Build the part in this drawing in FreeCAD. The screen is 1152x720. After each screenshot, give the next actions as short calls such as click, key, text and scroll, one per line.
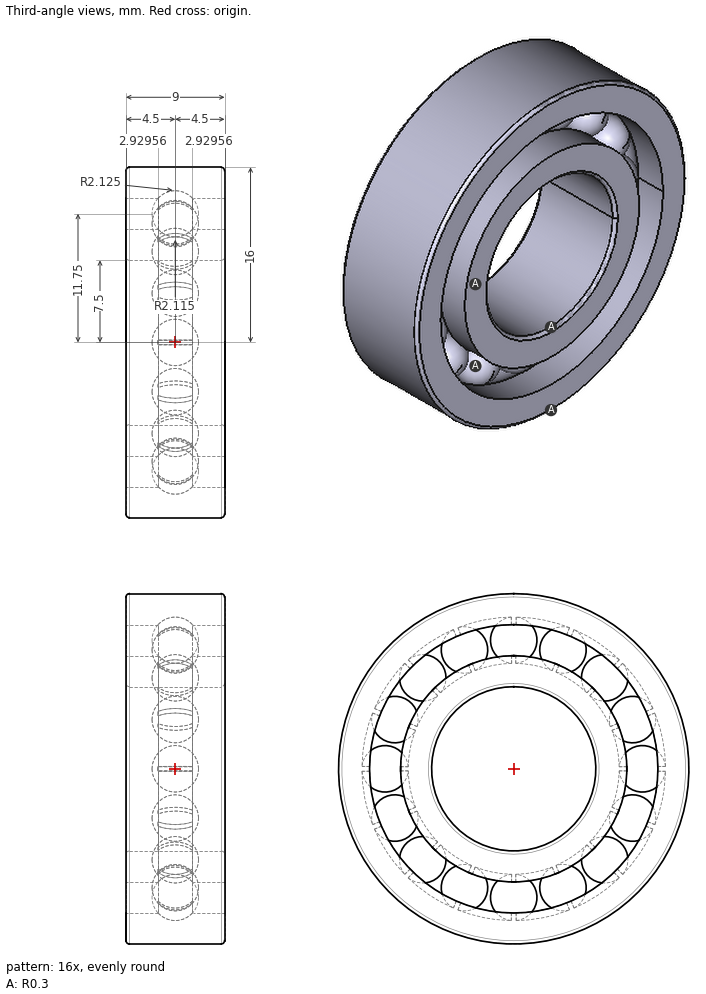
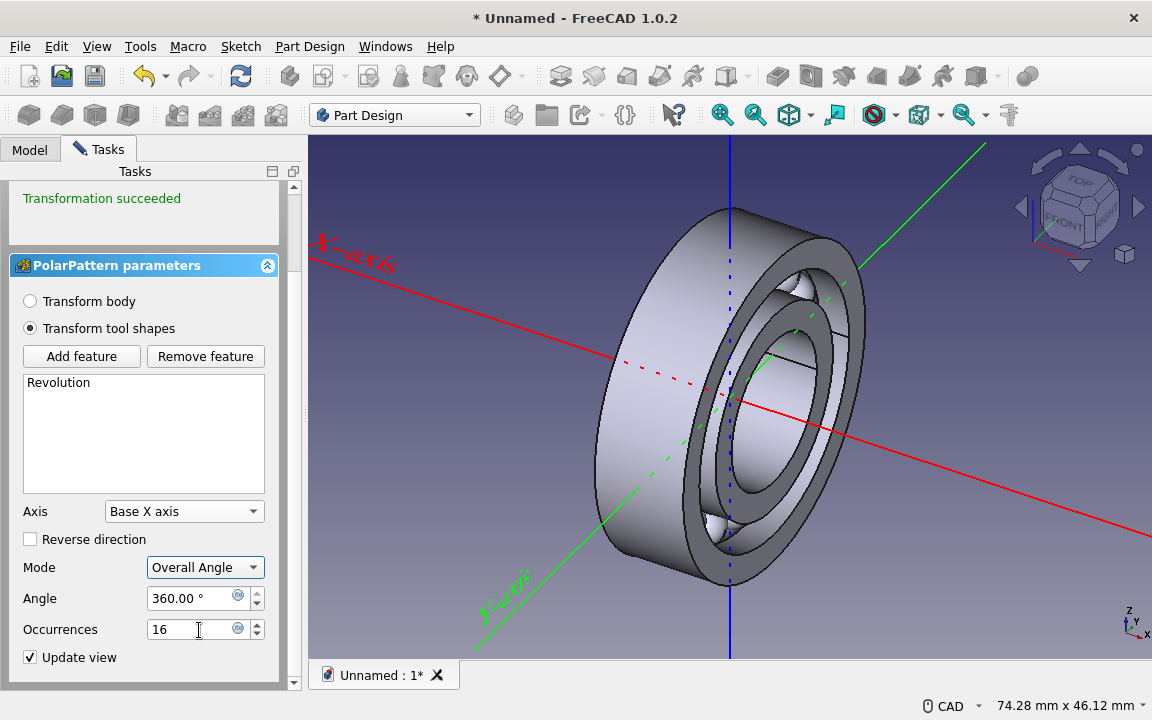
scroll(294, 436, up, 3)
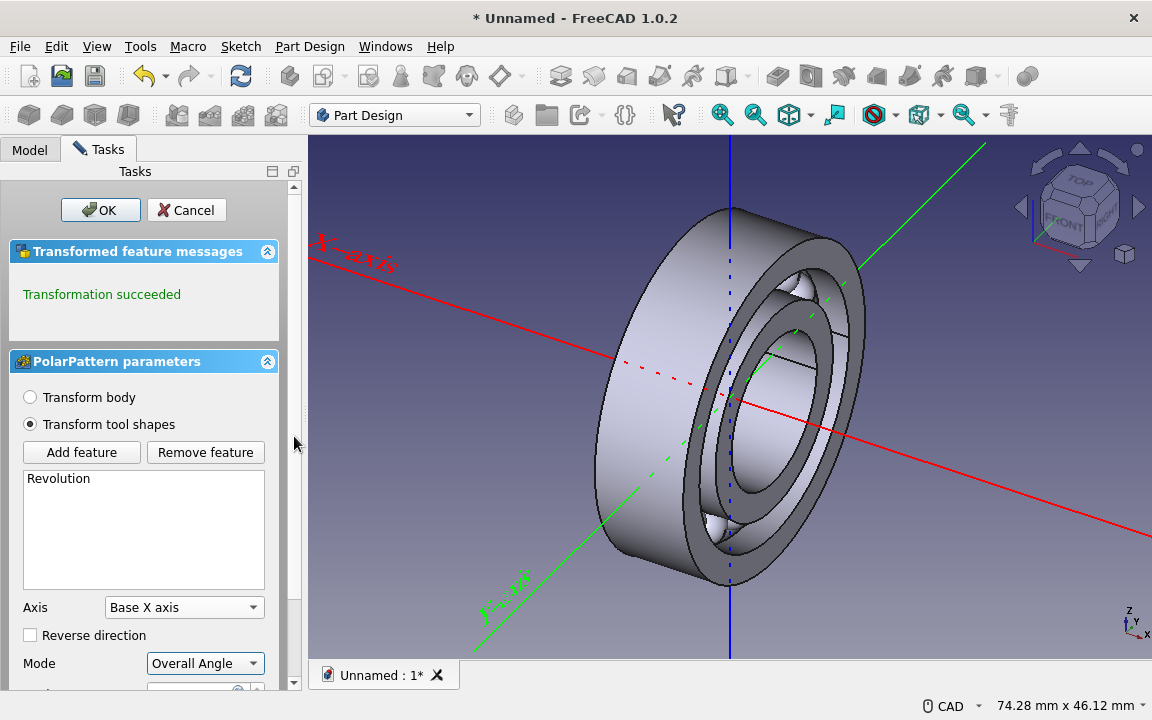
click(101, 210)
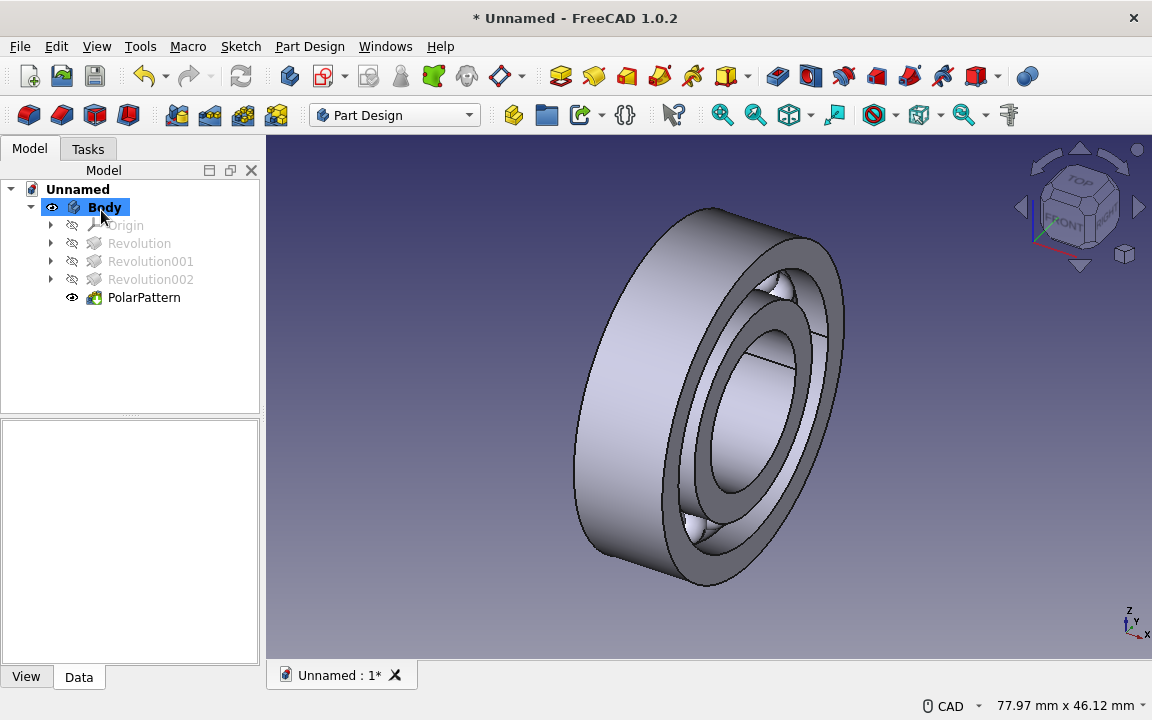
click(662, 501)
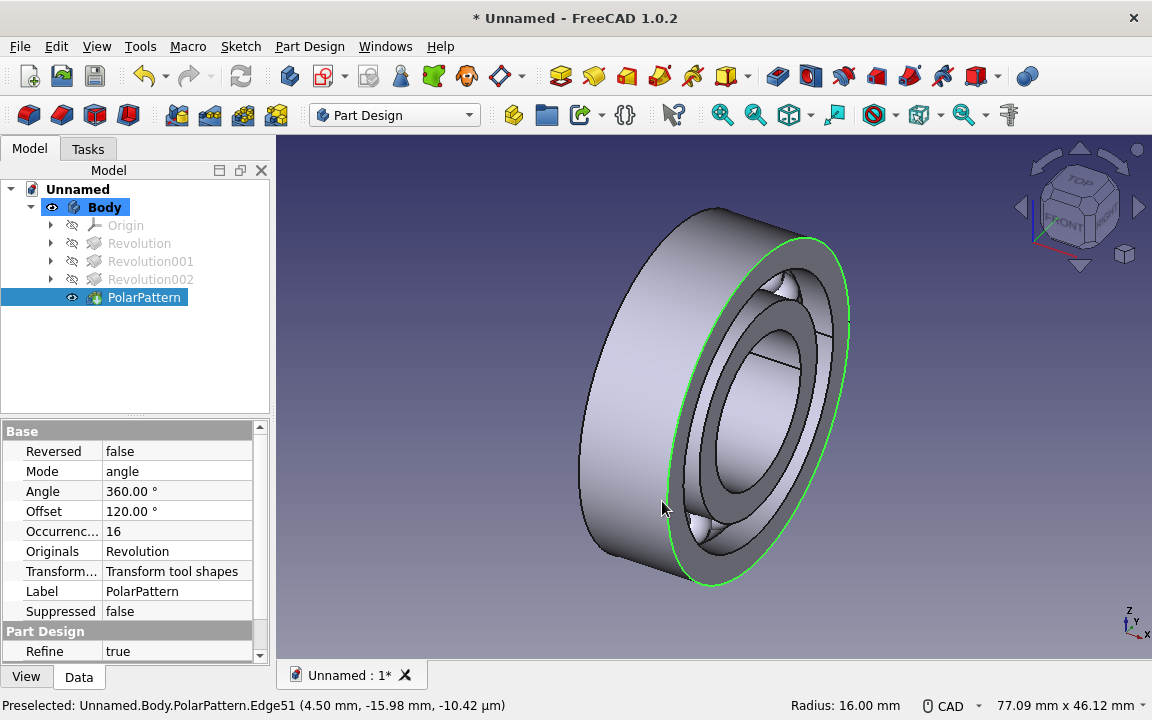
click(745, 490, ctrl)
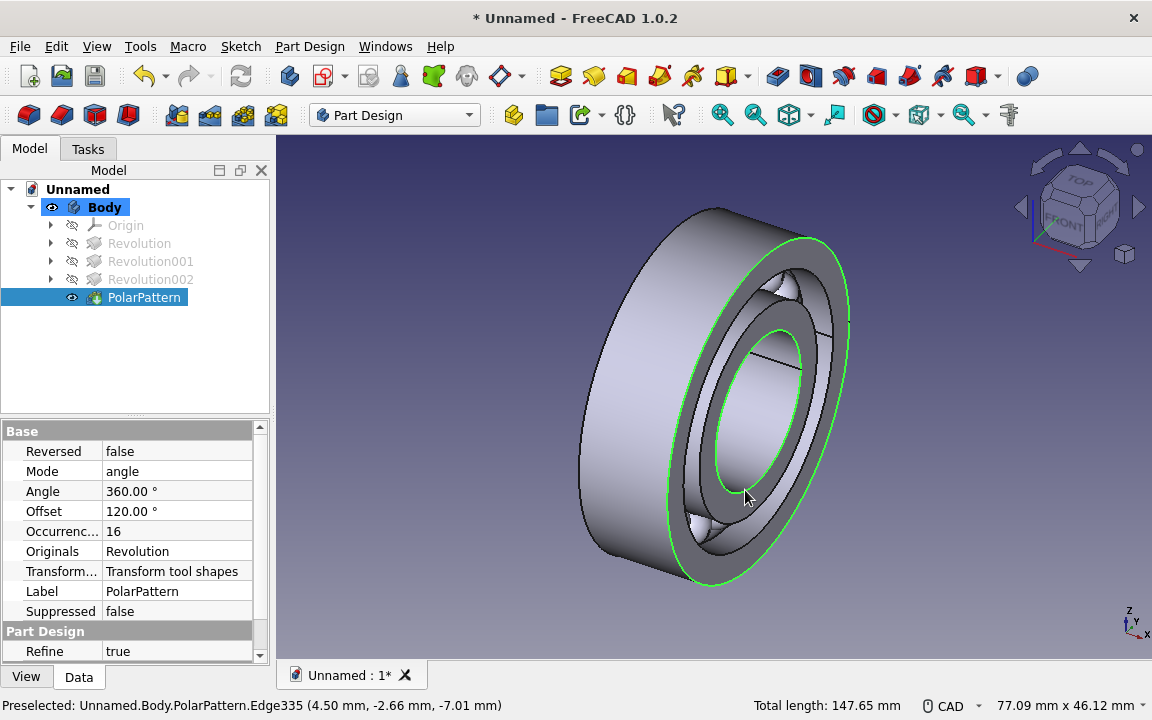
key(0)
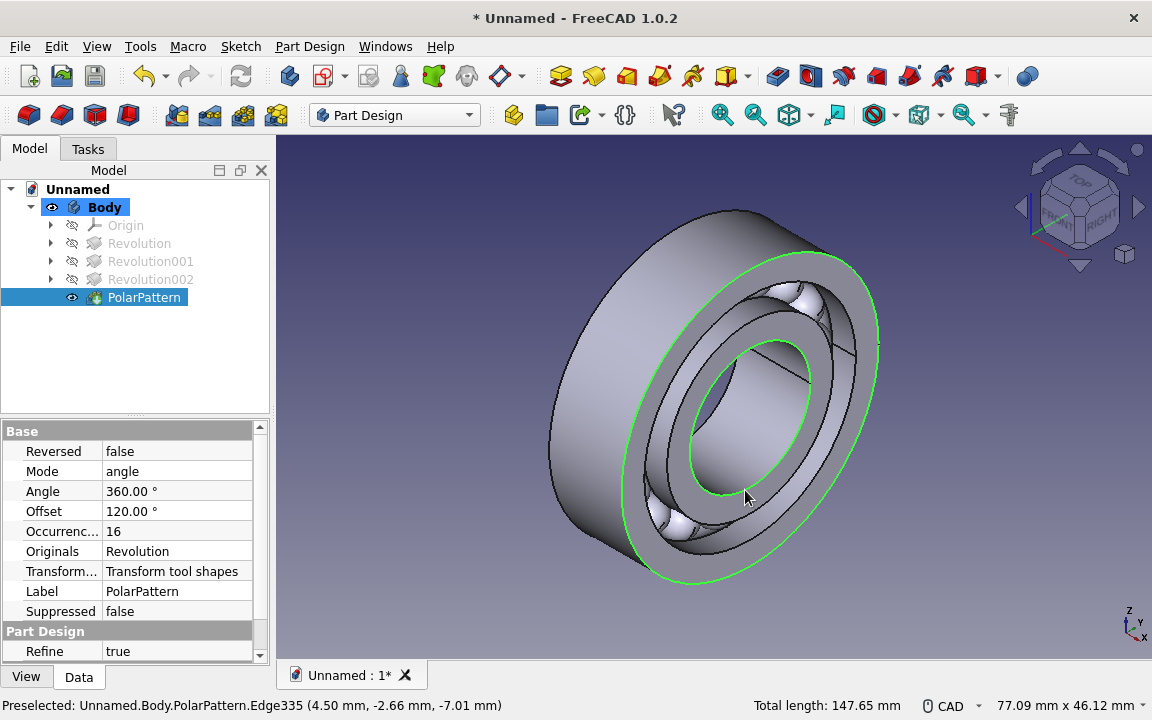
key(2)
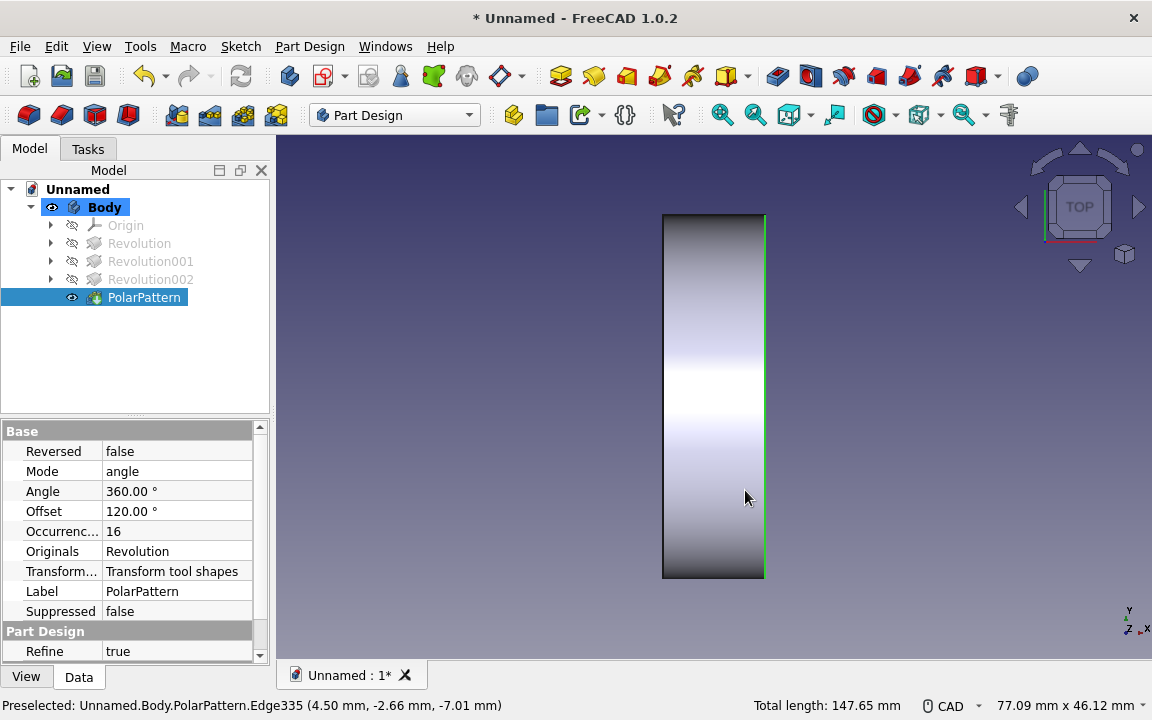
click(663, 543, ctrl)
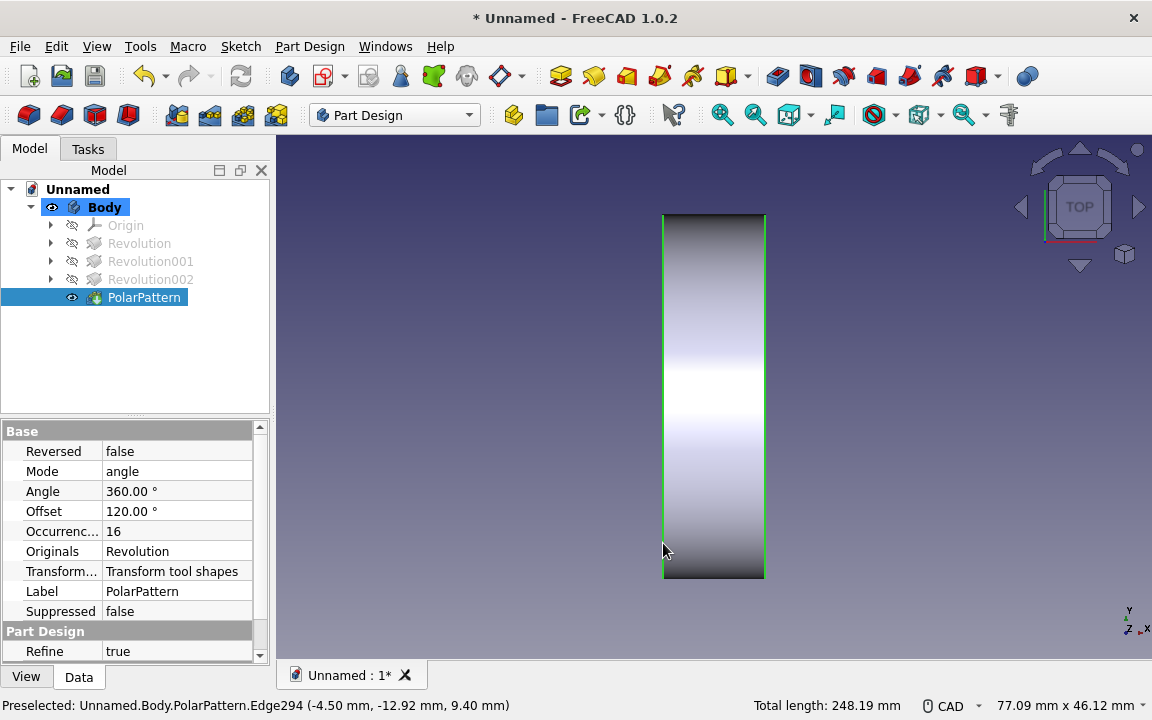
key(1)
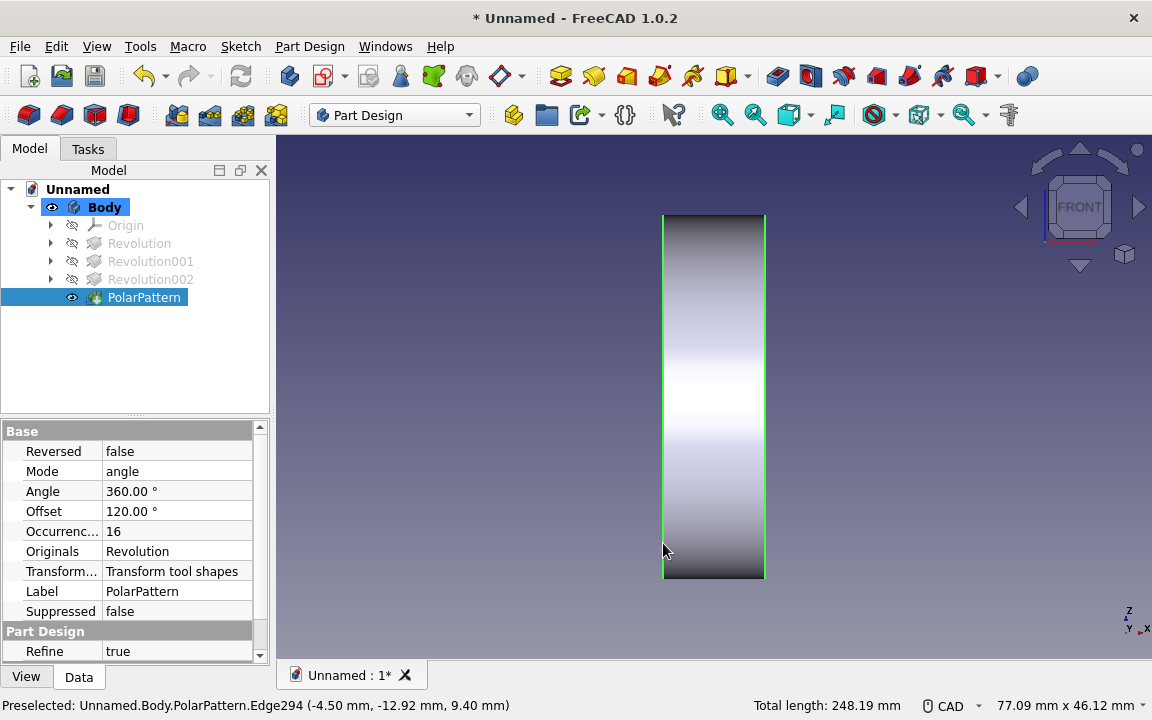
key(3)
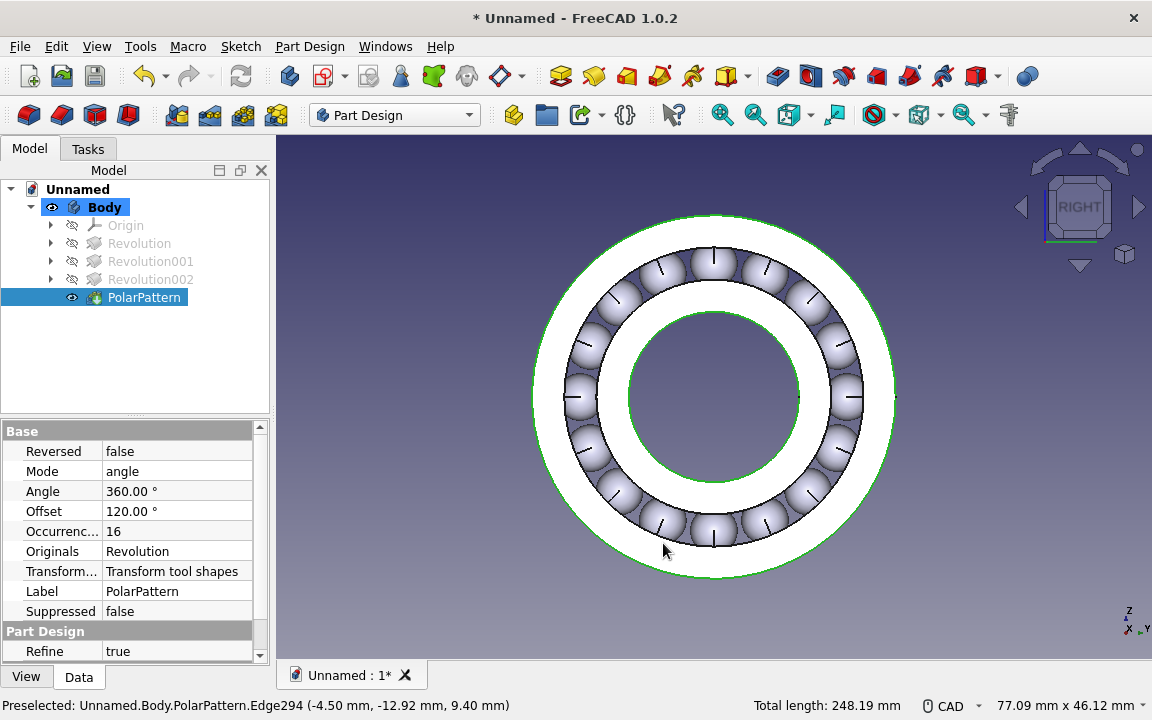
key(5)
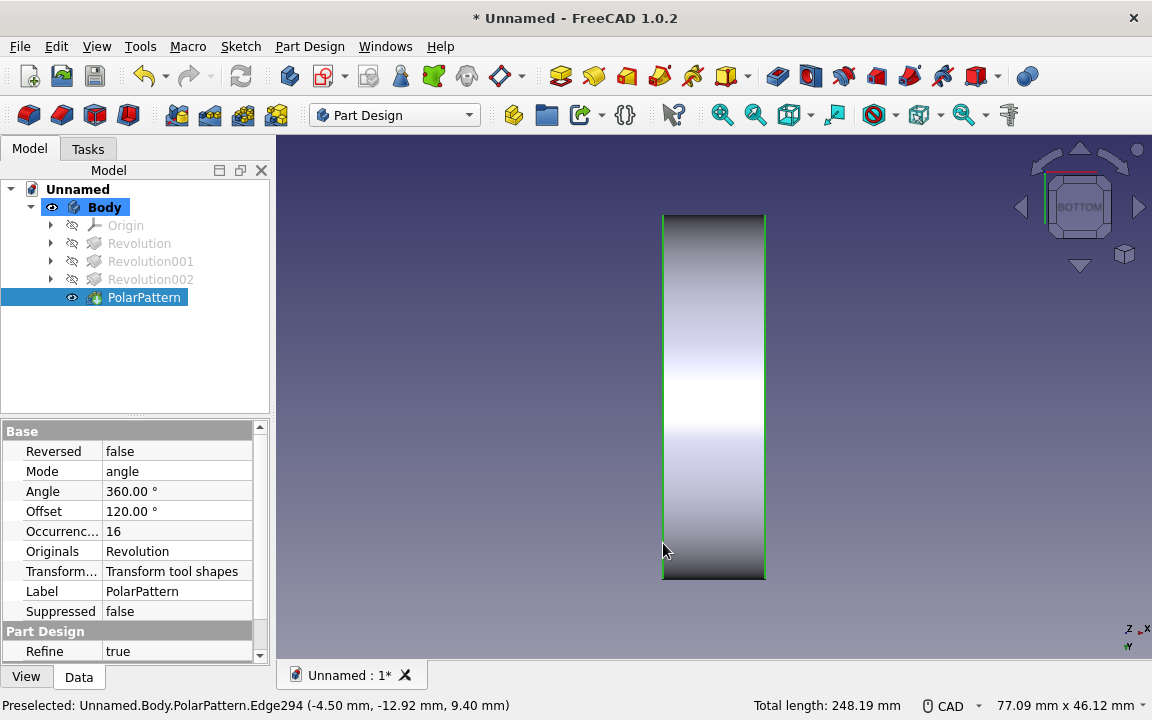
key(4)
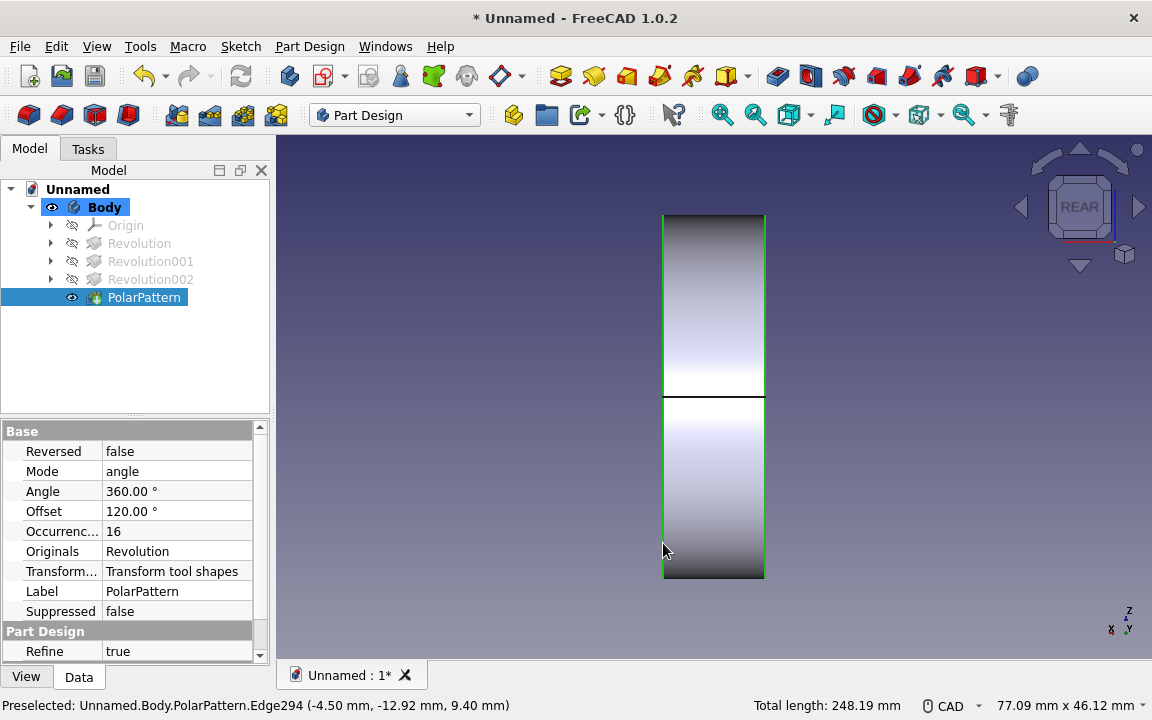
key(6)